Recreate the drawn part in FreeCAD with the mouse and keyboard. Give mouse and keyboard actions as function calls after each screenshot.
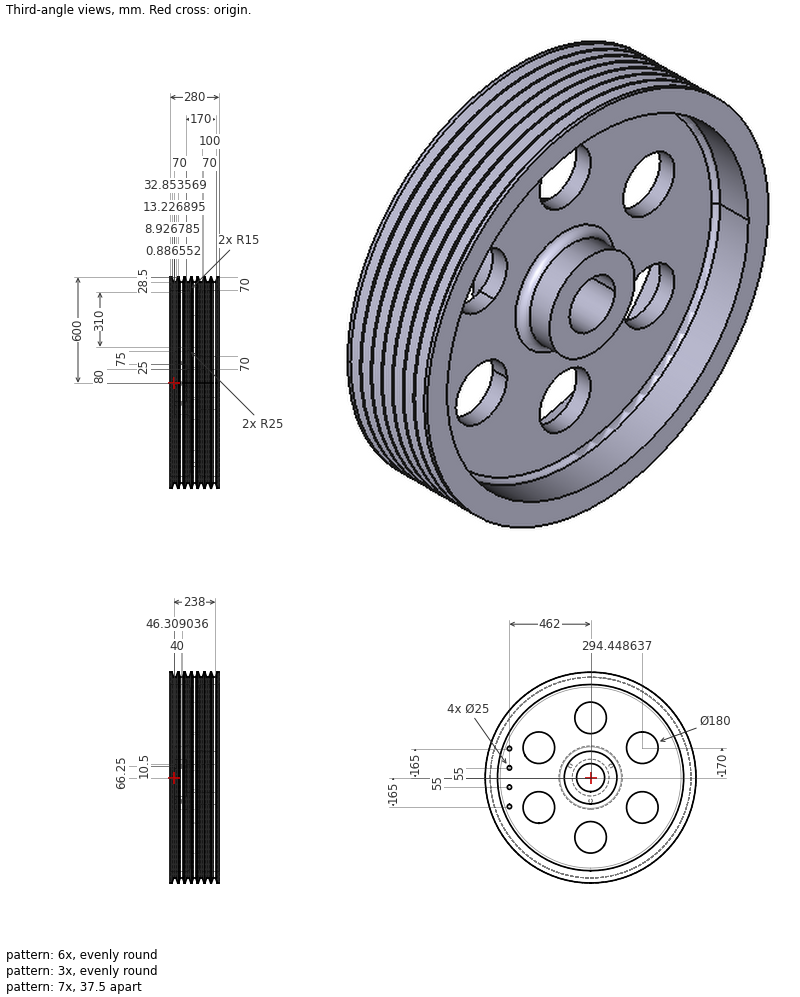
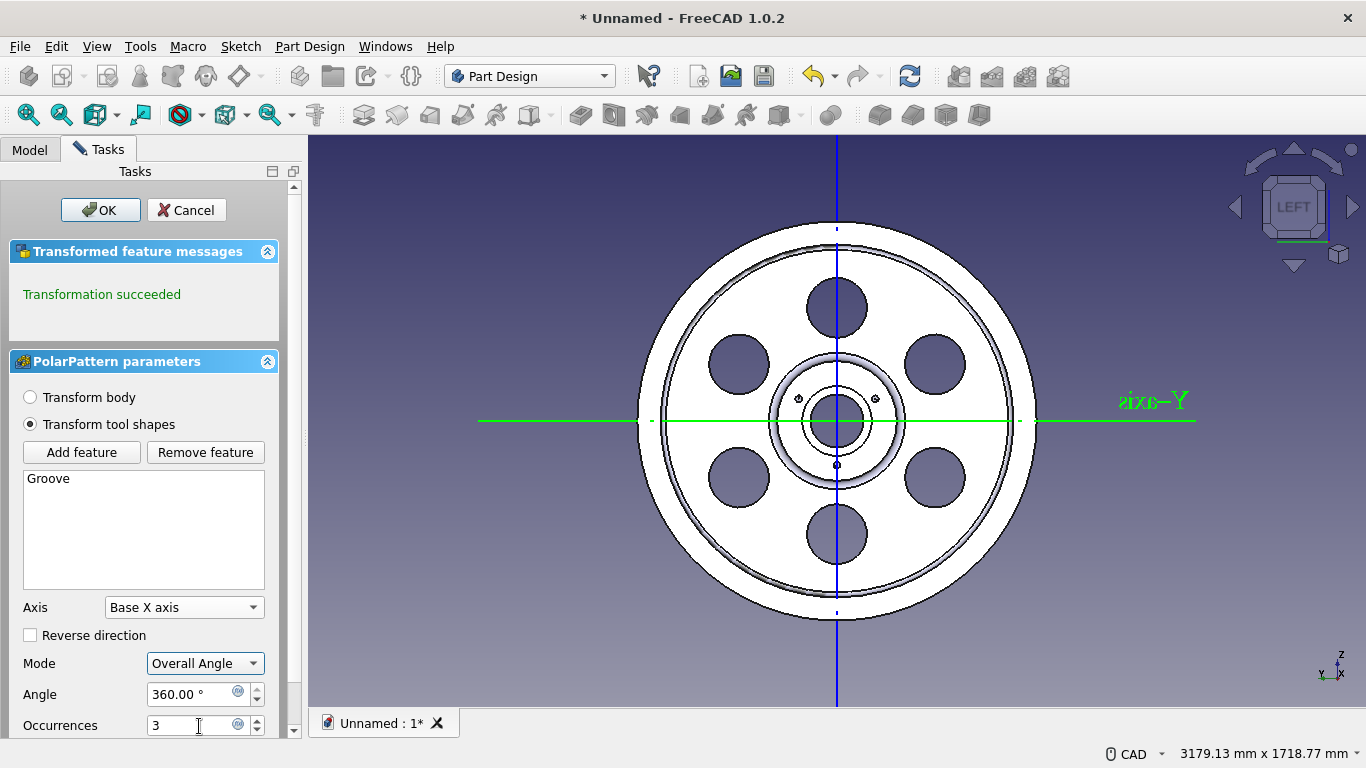
click(101, 210)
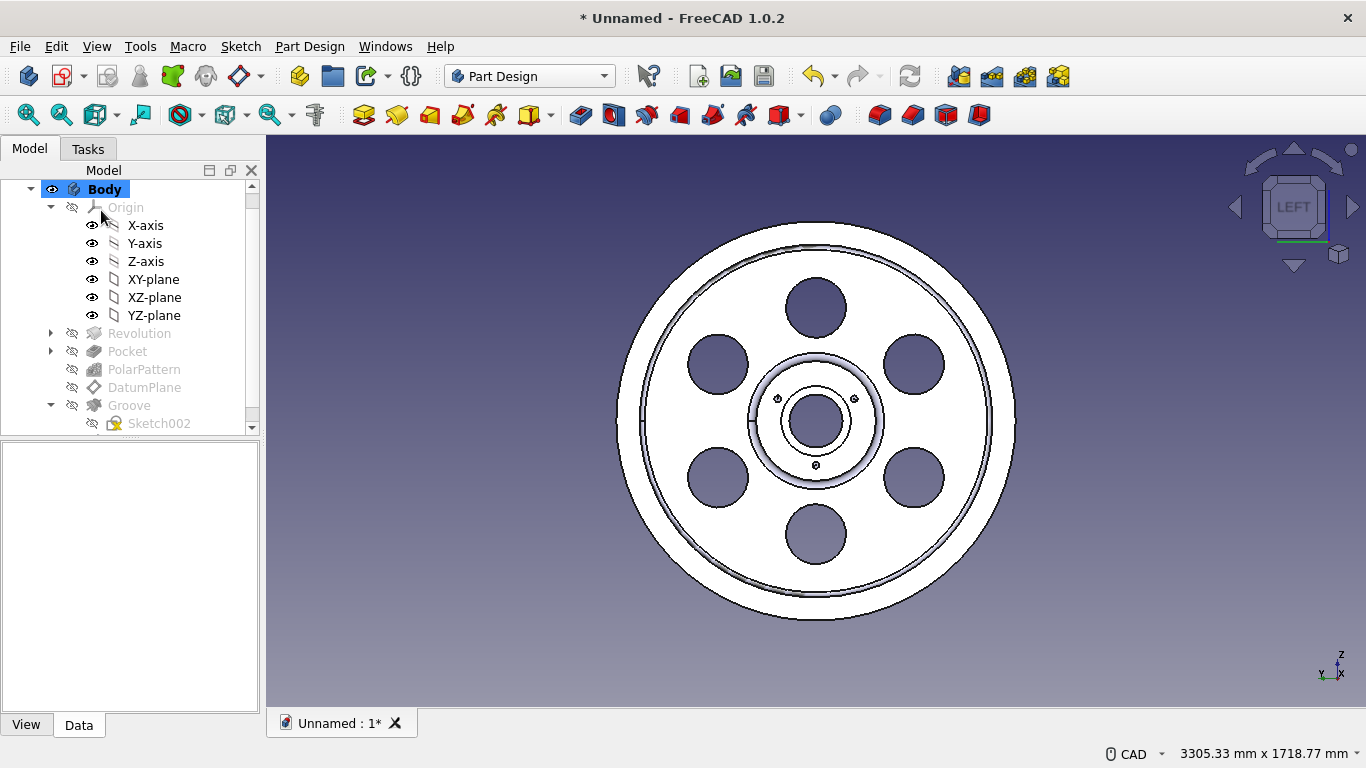
click(62, 76)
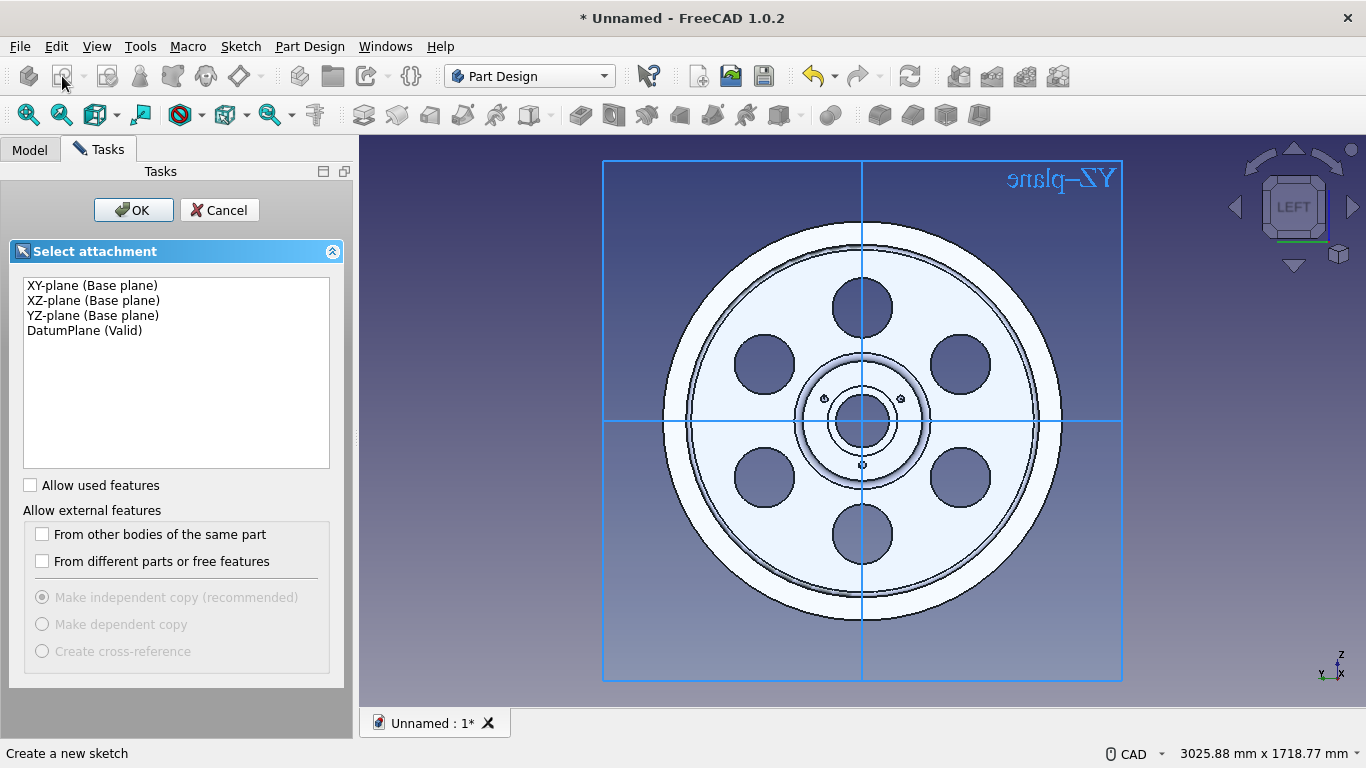
click(84, 316)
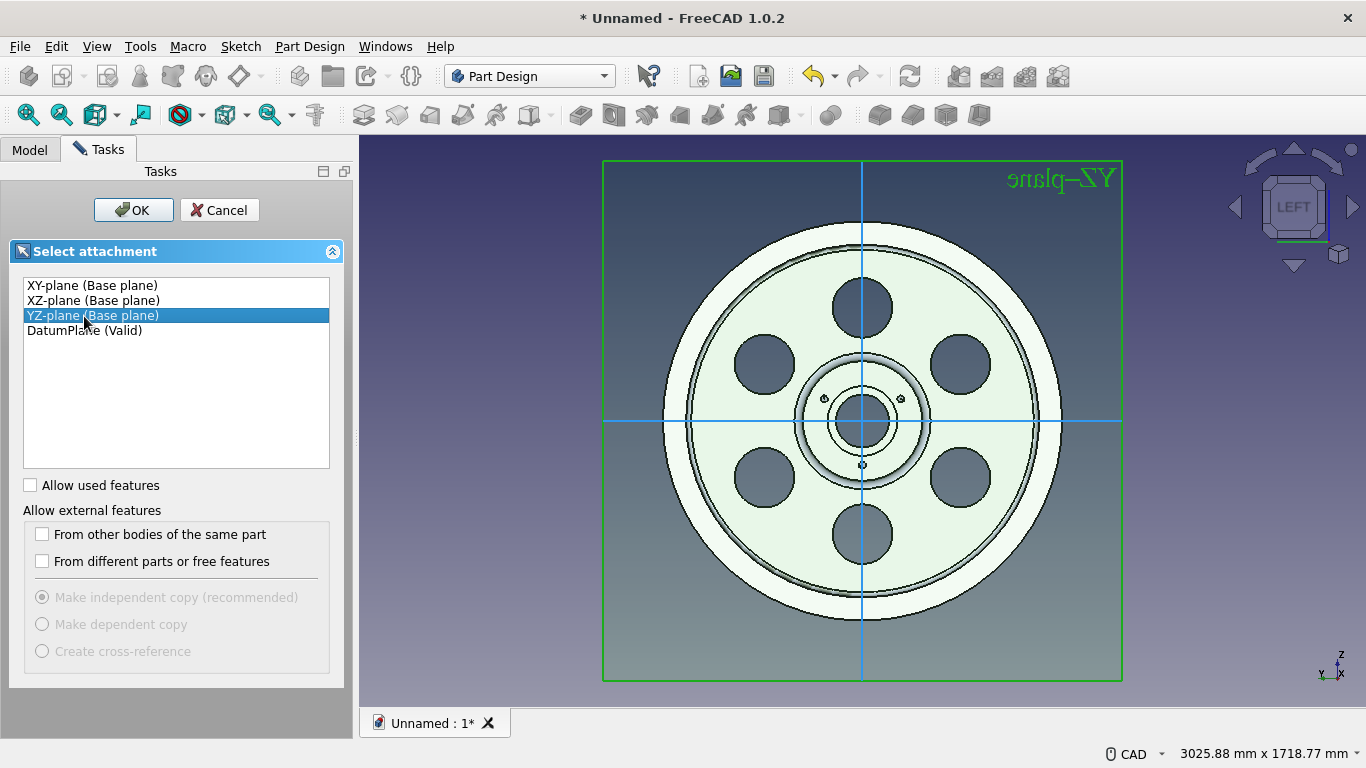
click(134, 210)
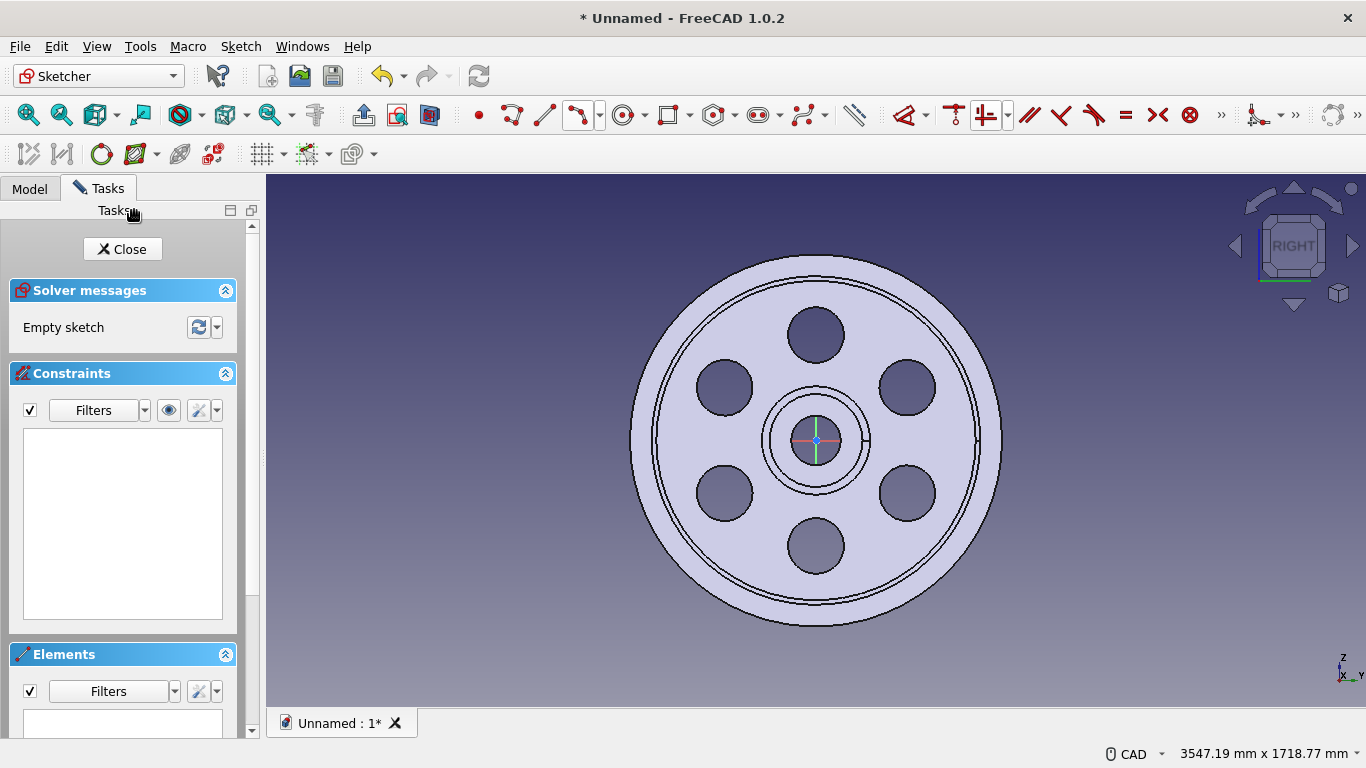
click(430, 116)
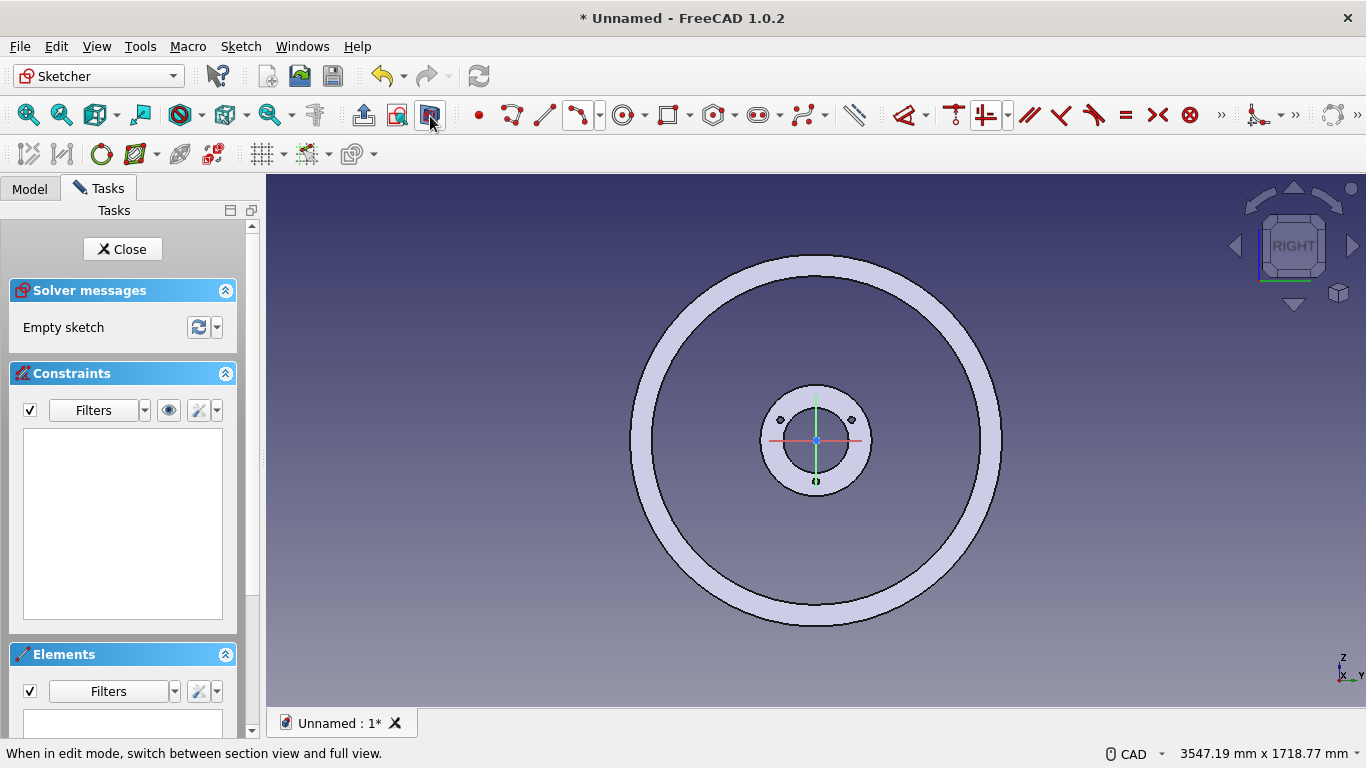
scroll(740, 441, up, 6)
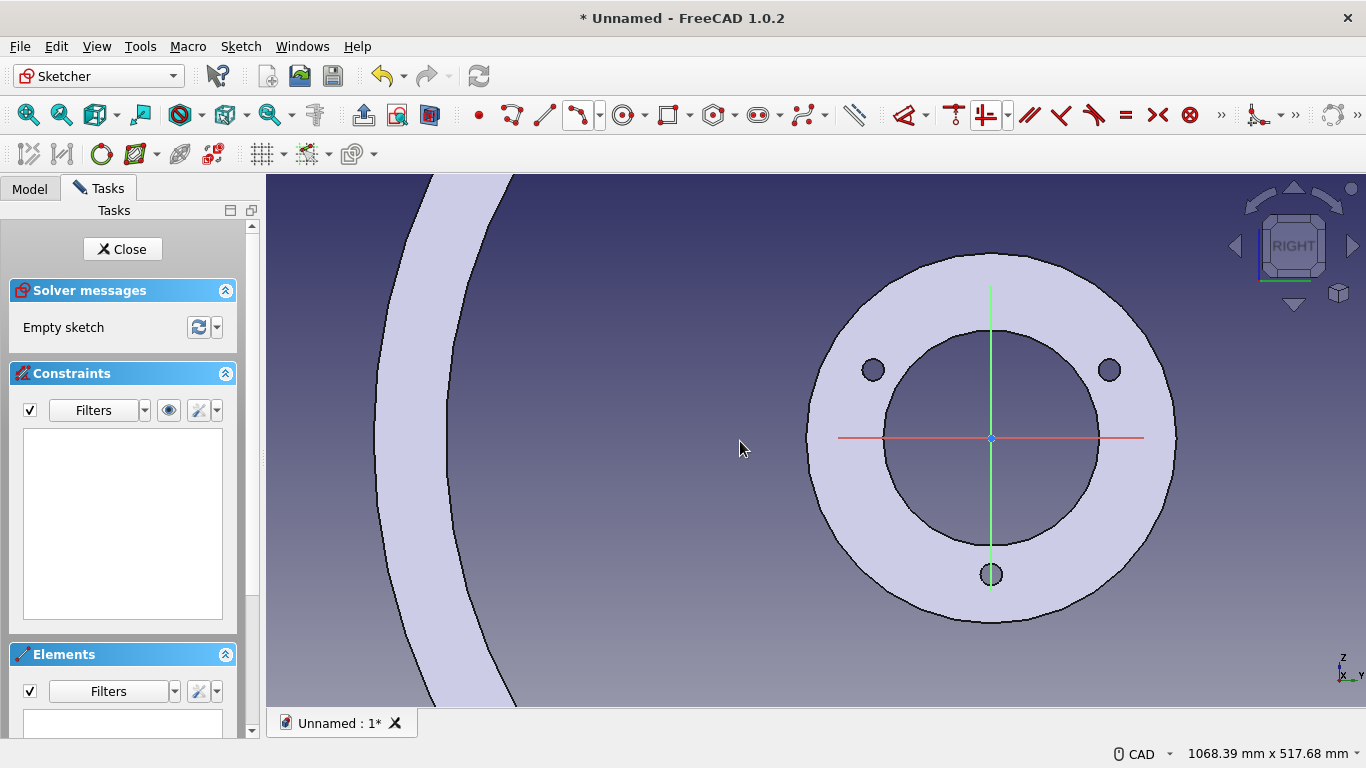
click(622, 116)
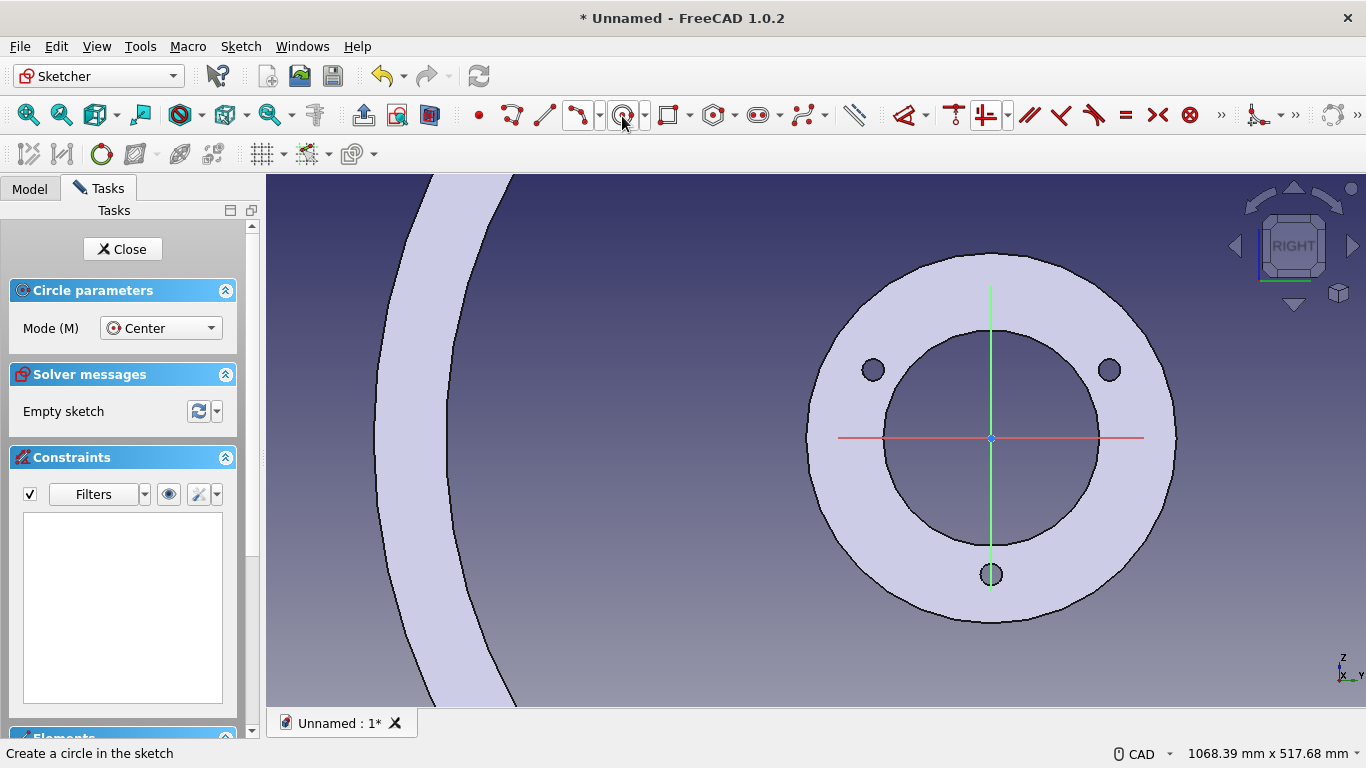
scroll(516, 382, up, 3)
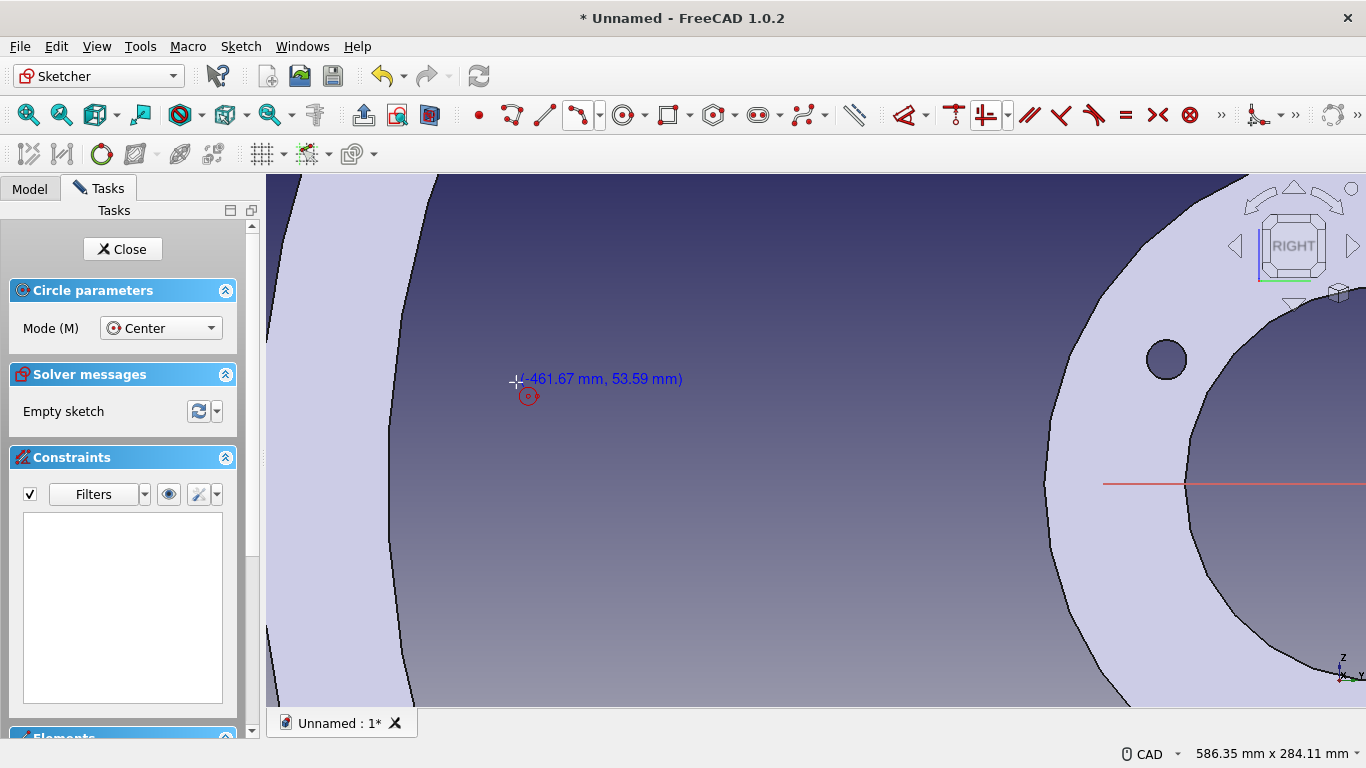
click(515, 381)
move(532, 364)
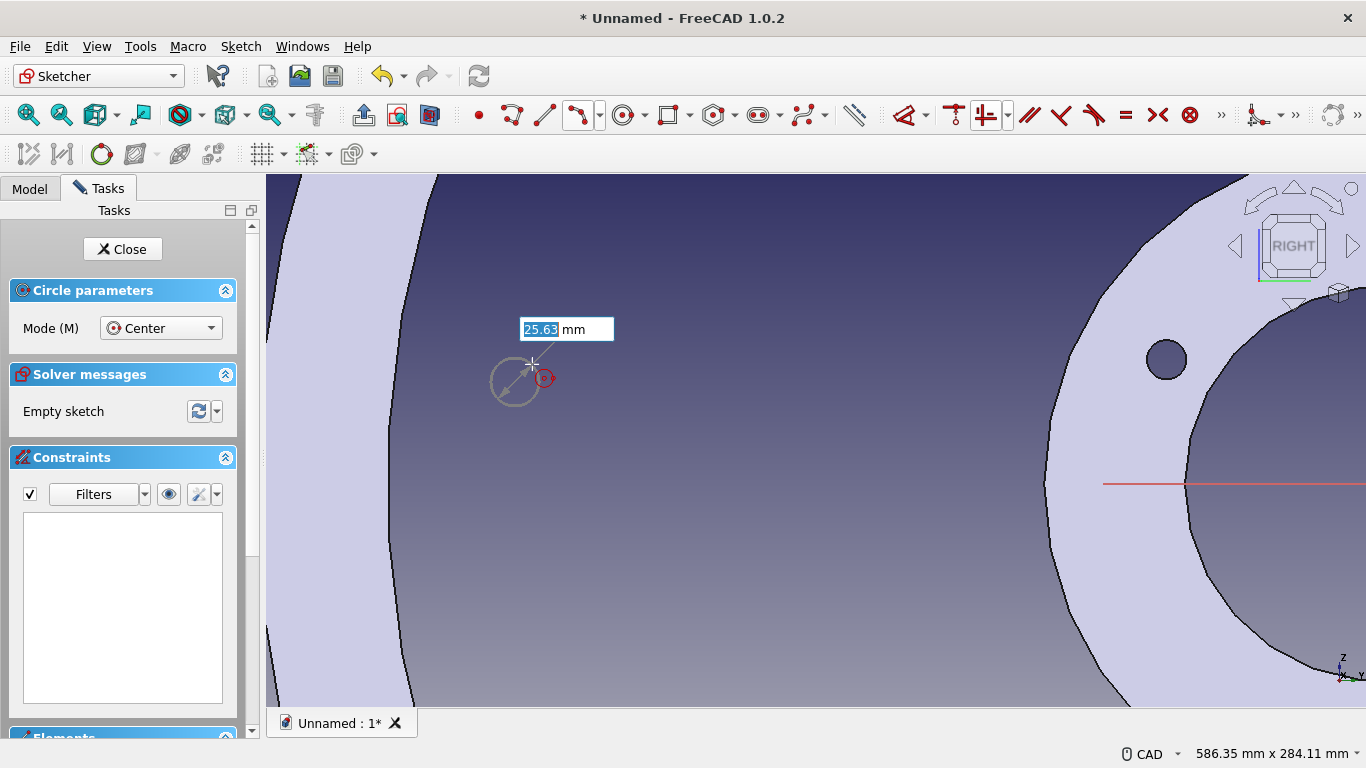
text(25)
key(Return)